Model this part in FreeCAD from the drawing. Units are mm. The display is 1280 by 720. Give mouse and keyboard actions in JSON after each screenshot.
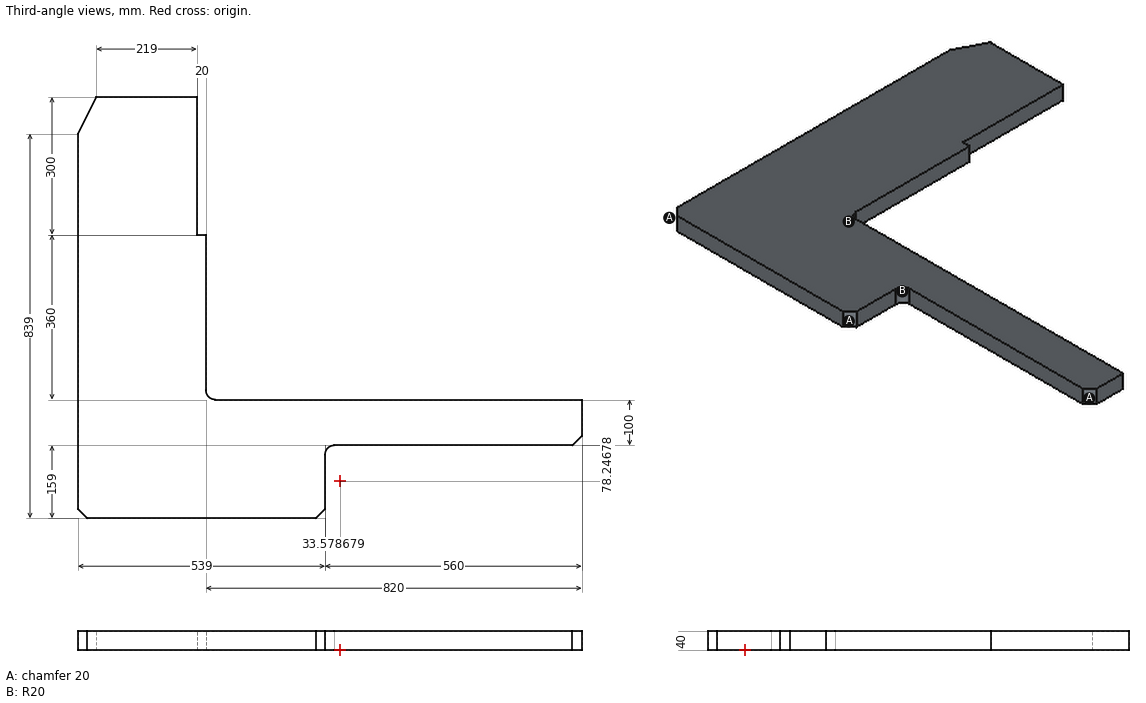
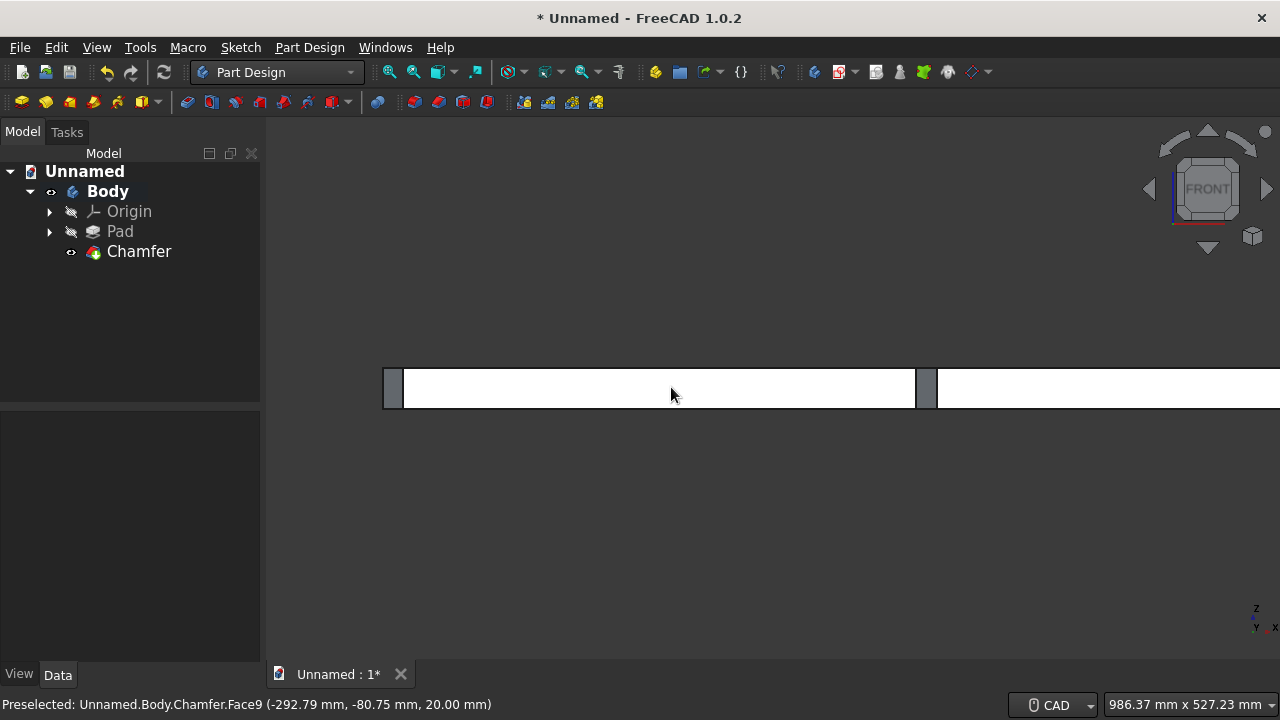
{"action": "key", "text": "v f"}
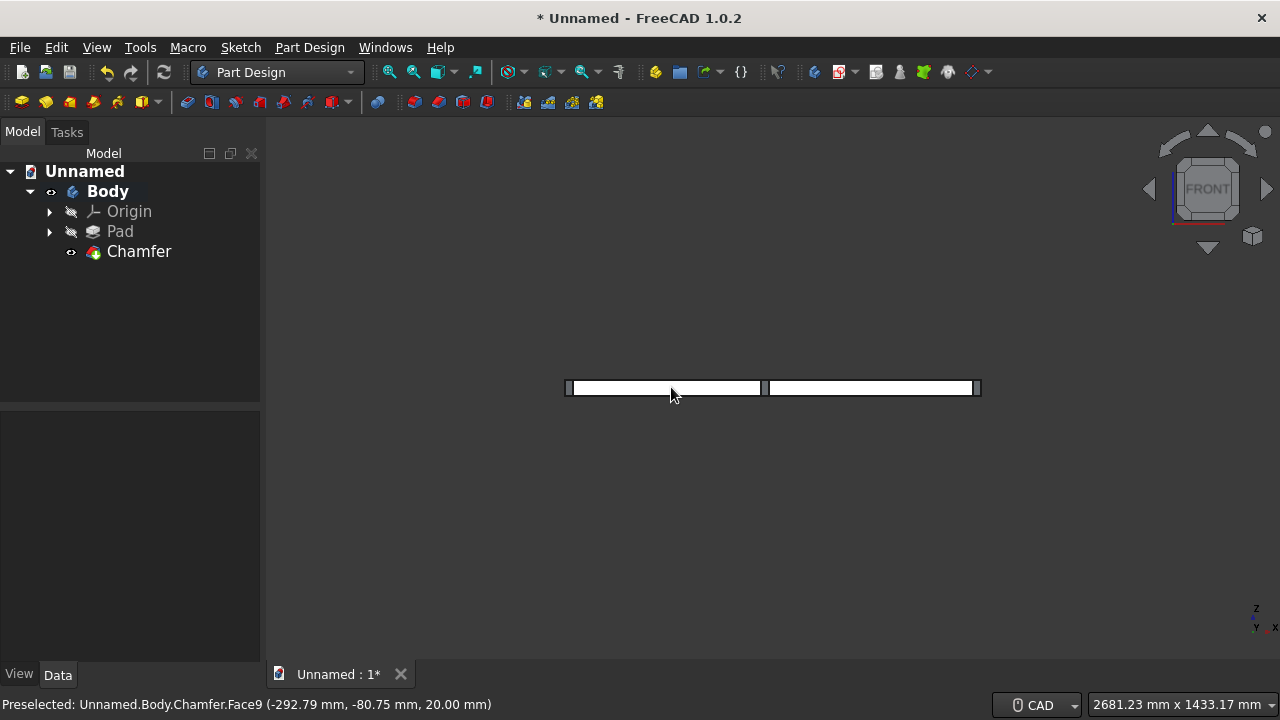
{"action": "key", "text": "0"}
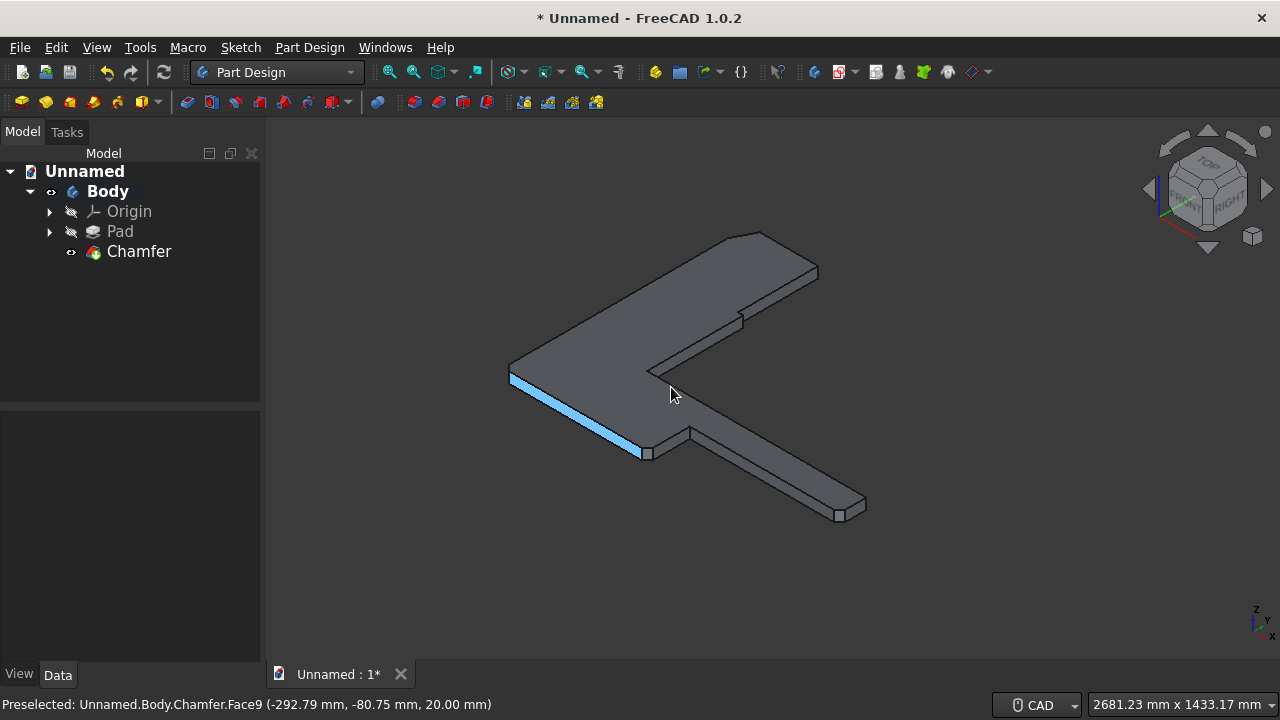
{"action": "scroll", "coordinate": [647, 376], "scroll_direction": "up", "scroll_amount": 5}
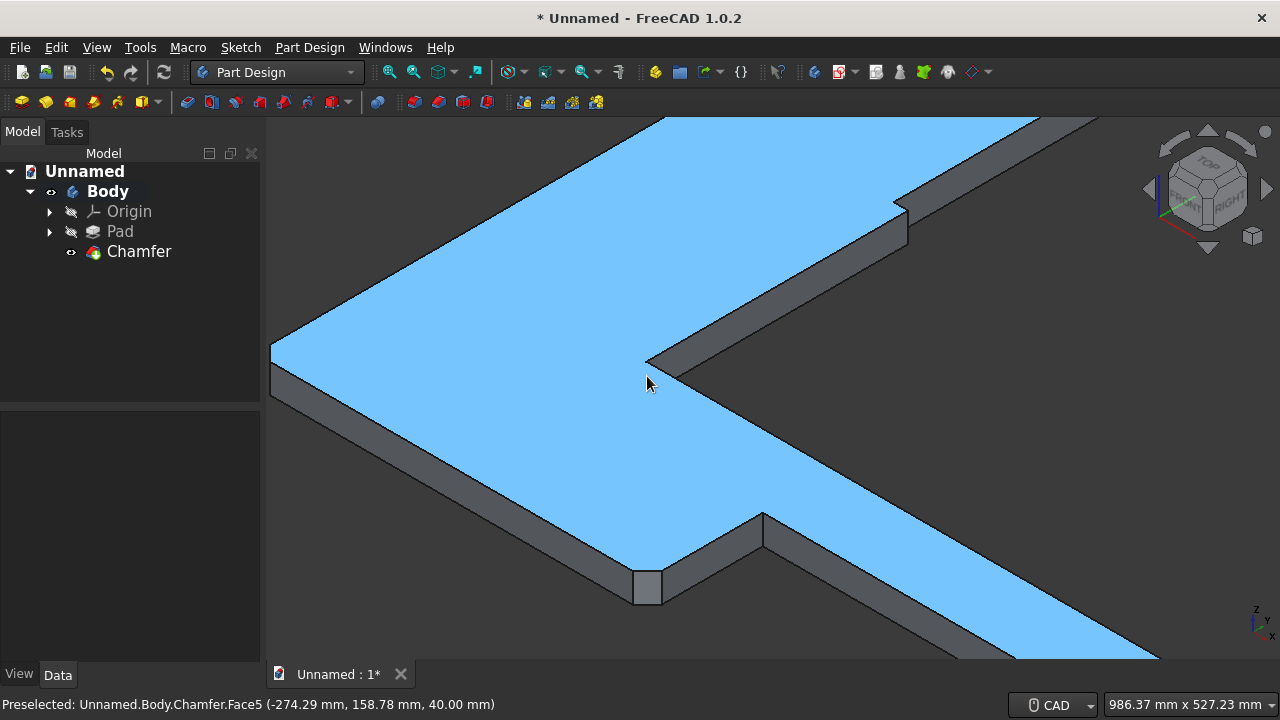
{"action": "key", "text": "v f"}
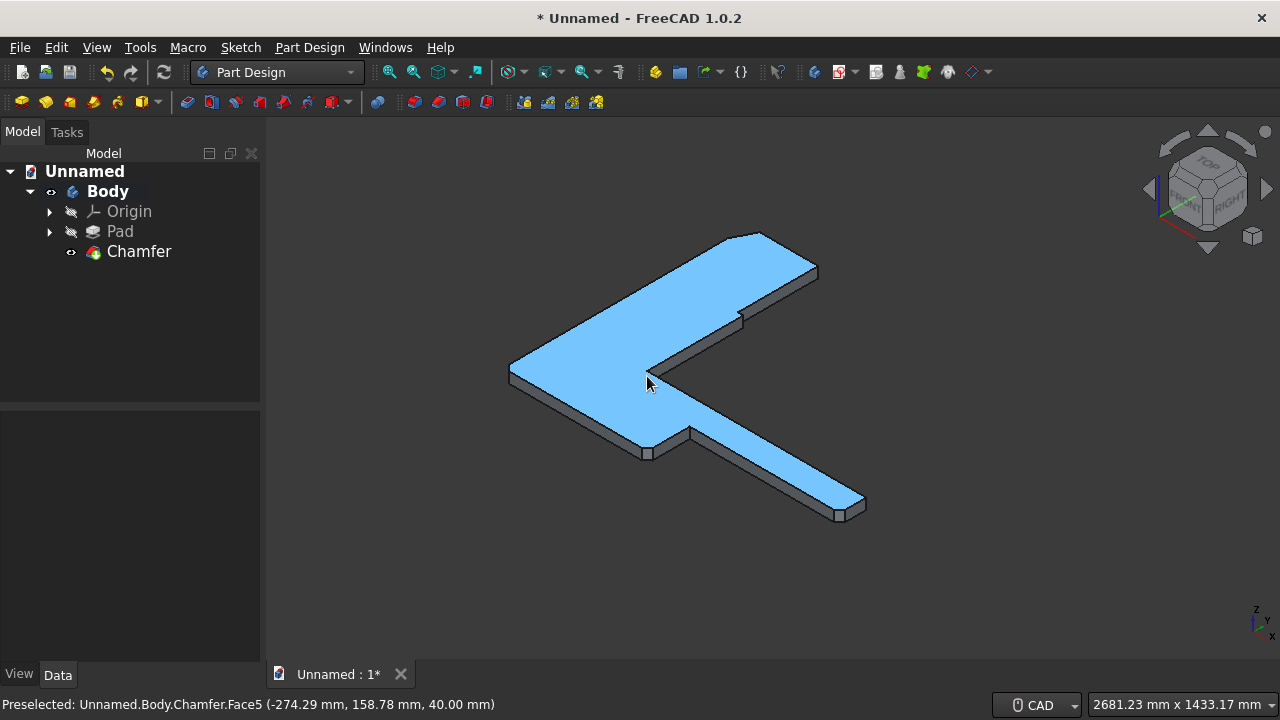
{"action": "key", "text": "2"}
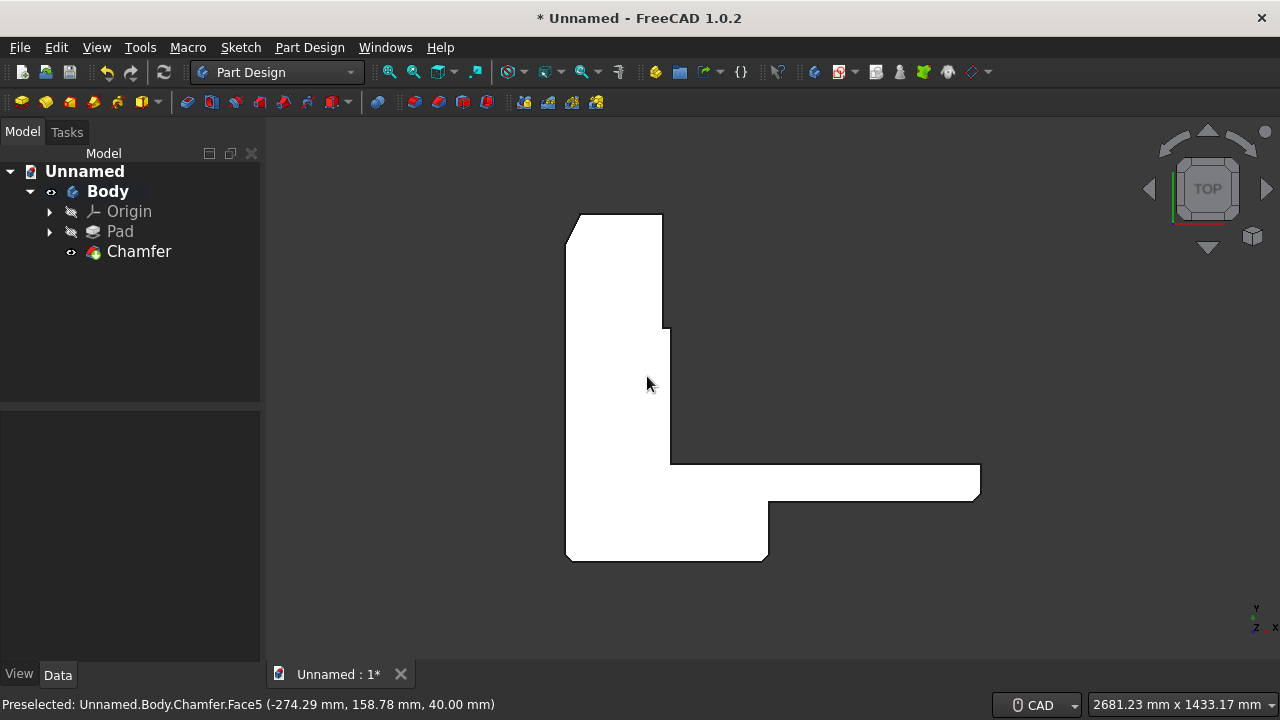
{"action": "scroll", "coordinate": [671, 463], "scroll_direction": "up", "scroll_amount": 5}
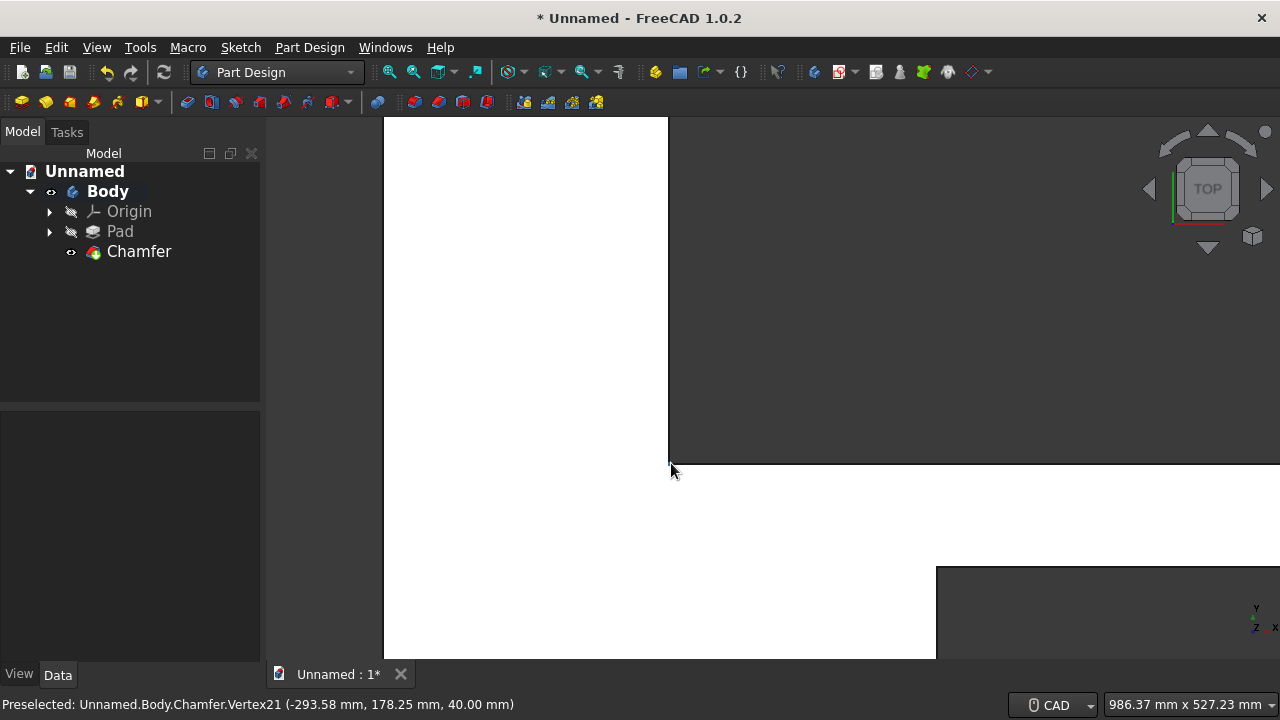
{"action": "left_click", "coordinate": [390, 72]}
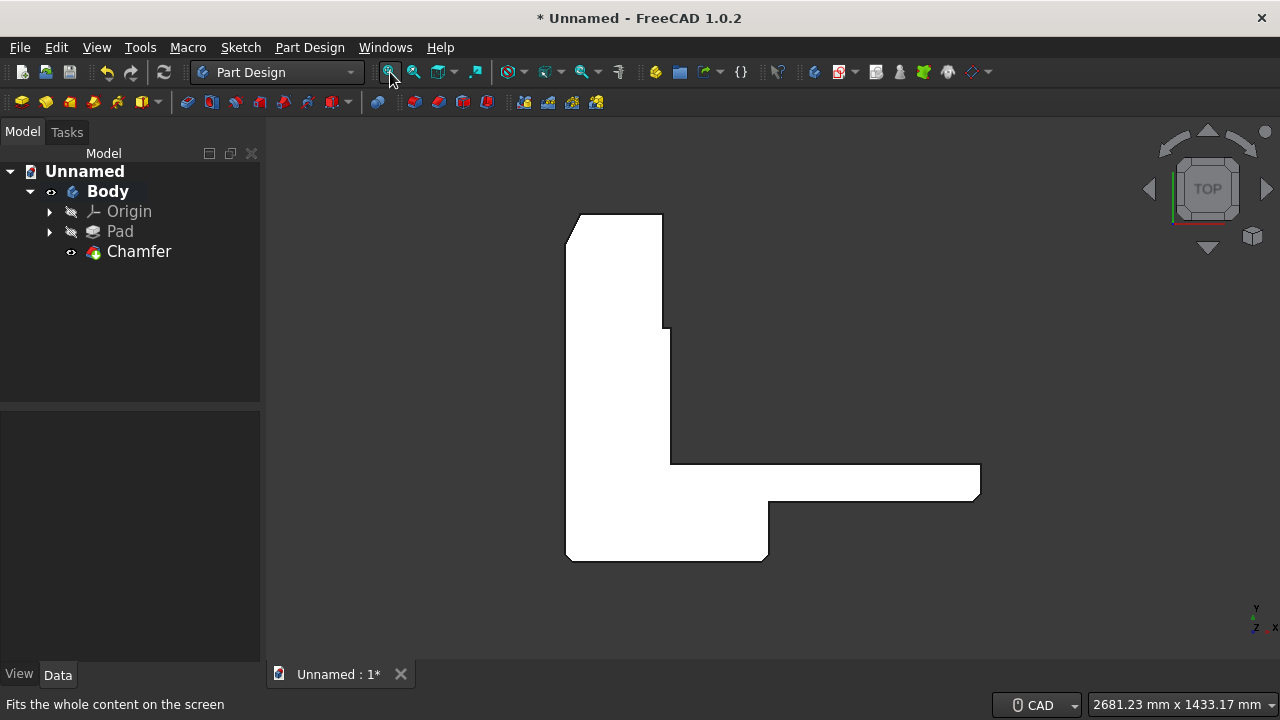
{"action": "key", "text": "1"}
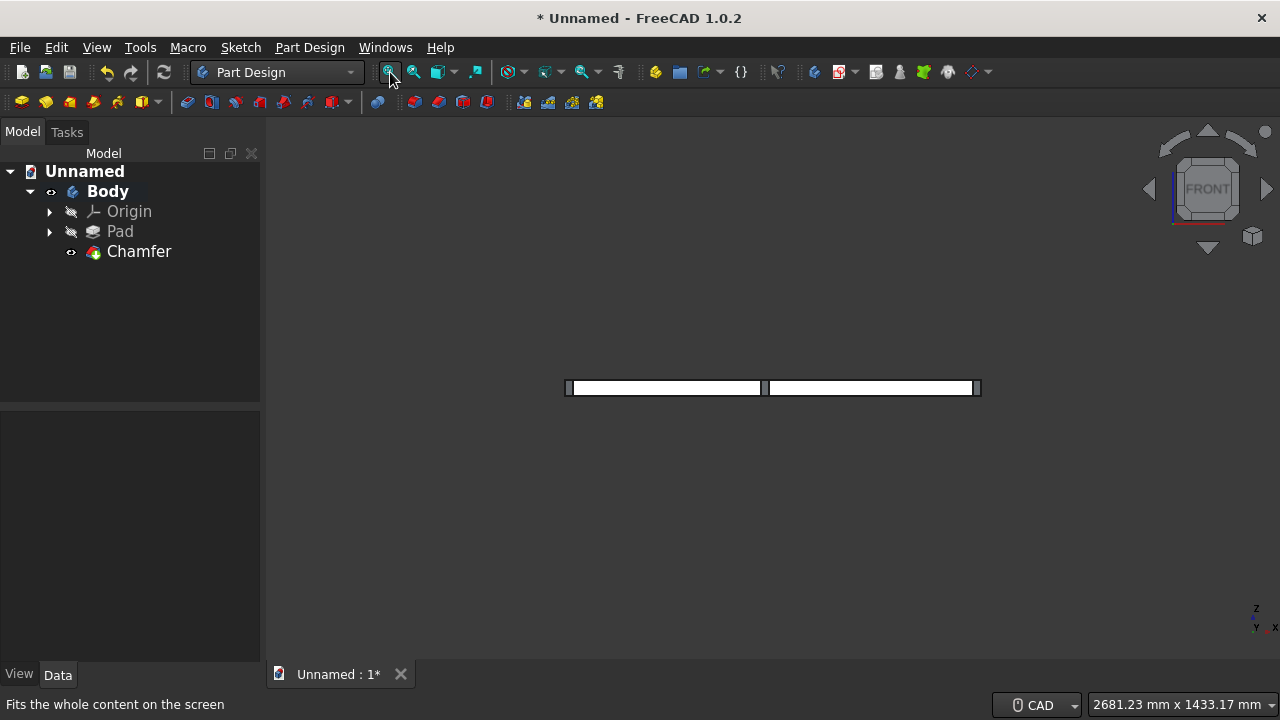
{"action": "left_click", "coordinate": [390, 72]}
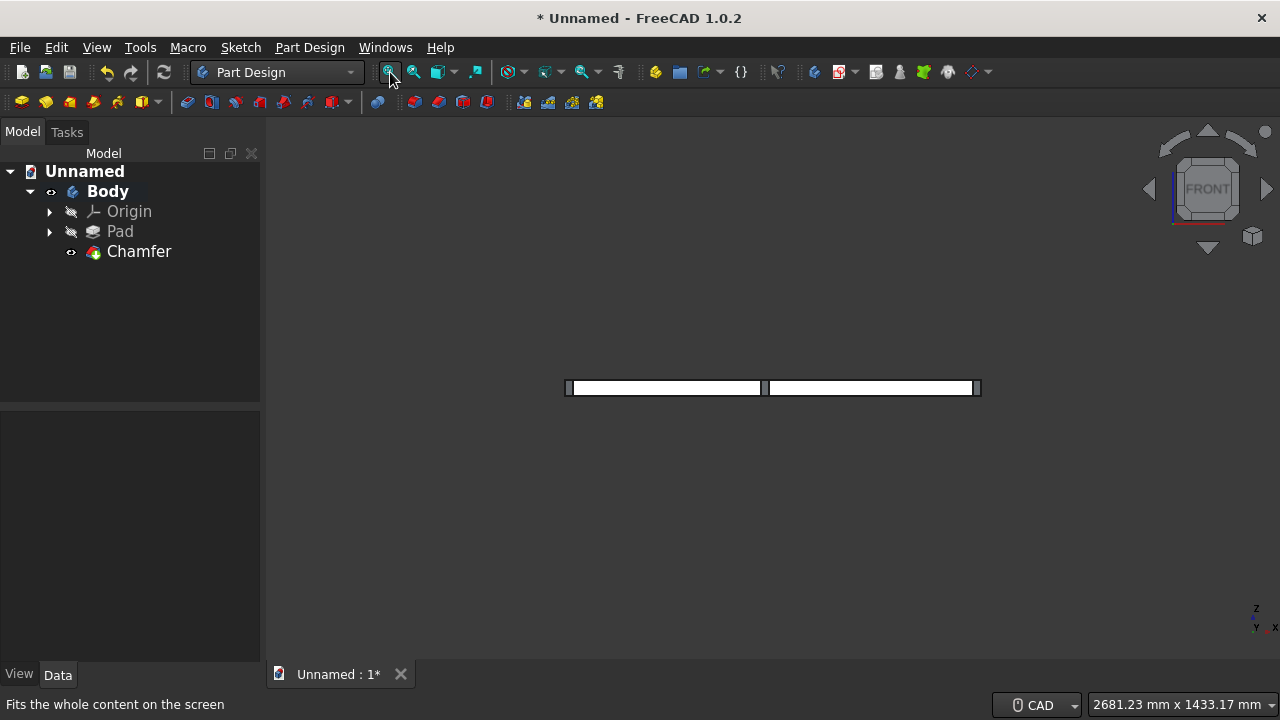
{"action": "scroll", "coordinate": [671, 387], "scroll_direction": "up", "scroll_amount": 5}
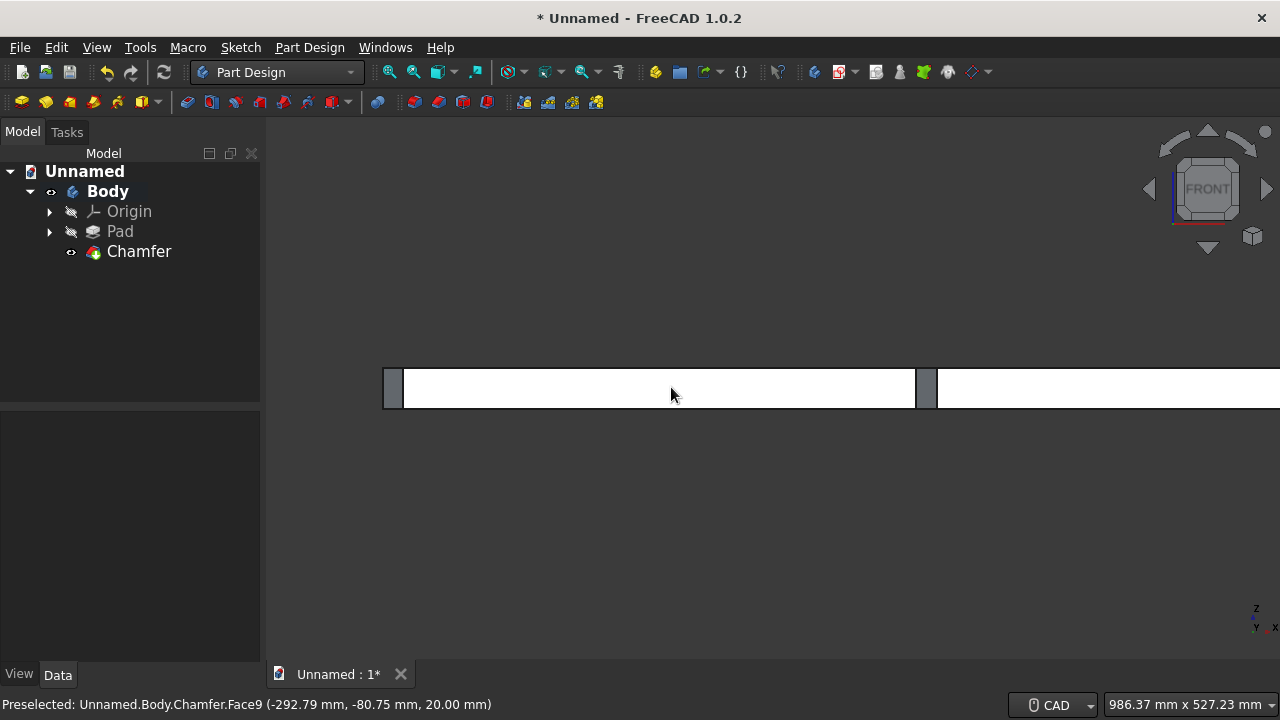
{"action": "key", "text": "v f"}